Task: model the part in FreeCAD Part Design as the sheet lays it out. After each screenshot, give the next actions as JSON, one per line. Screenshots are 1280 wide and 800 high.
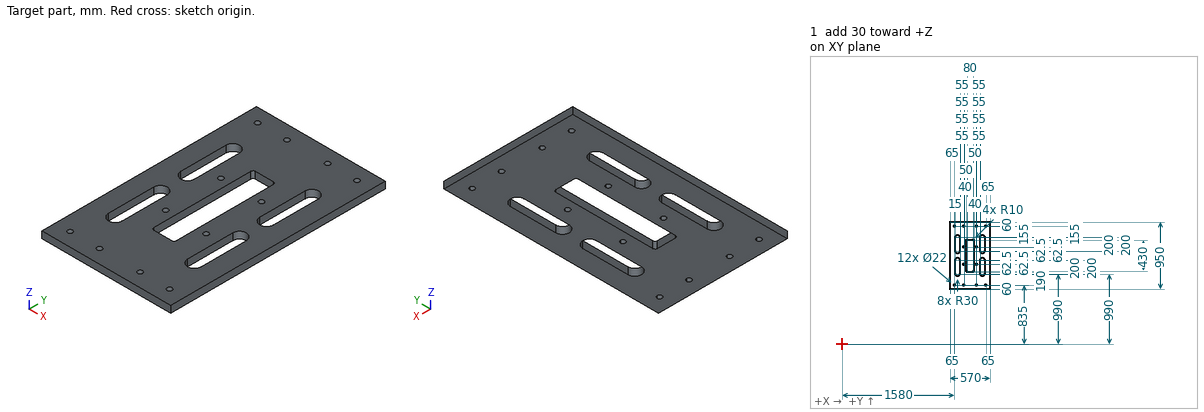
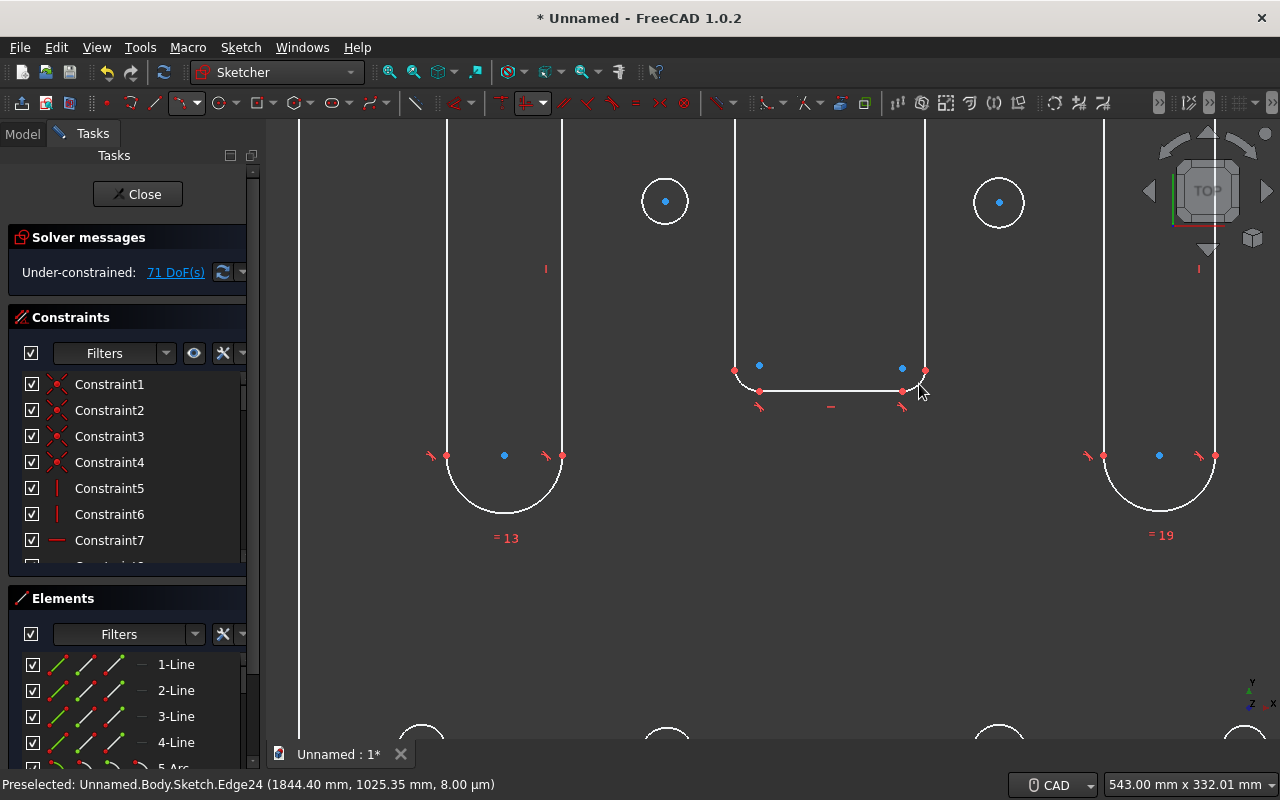
{"action": "scroll", "coordinate": [906, 388], "scroll_direction": "down", "scroll_amount": 10}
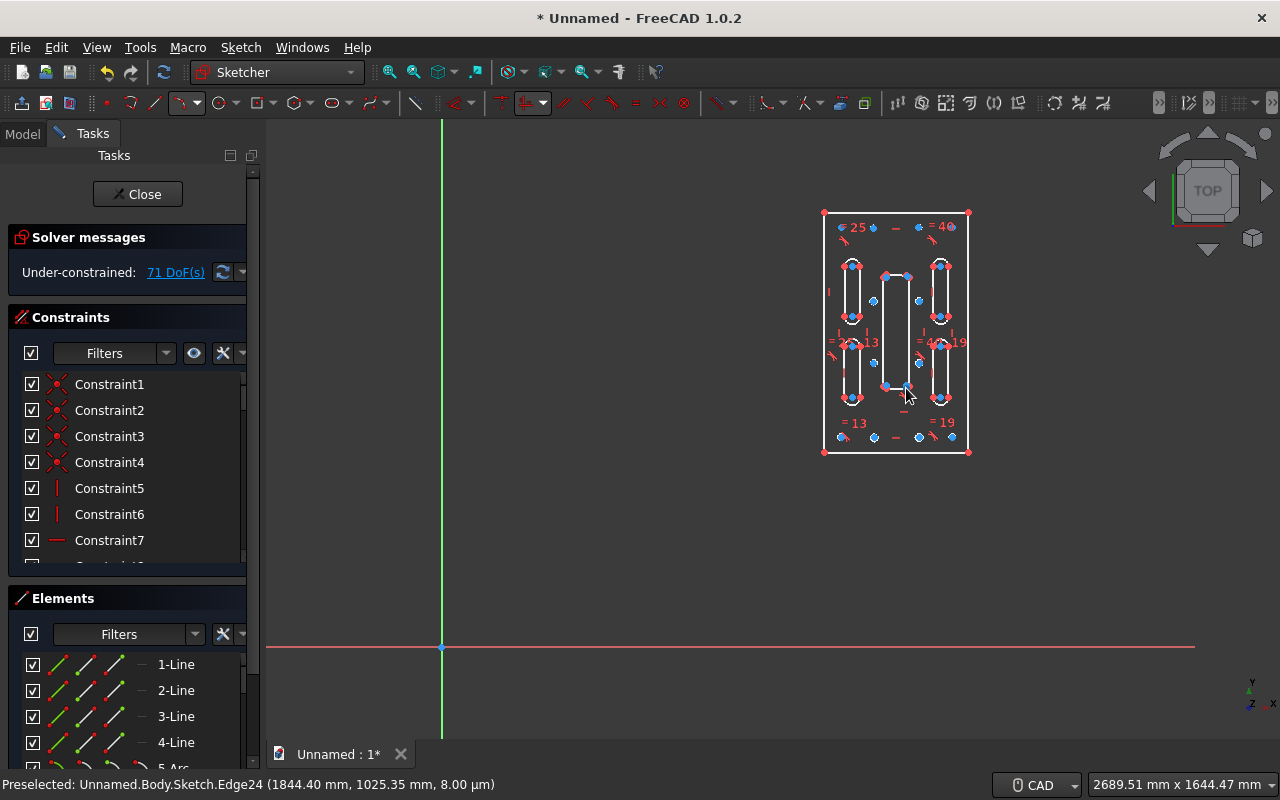
{"action": "scroll", "coordinate": [883, 364], "scroll_direction": "up", "scroll_amount": 4}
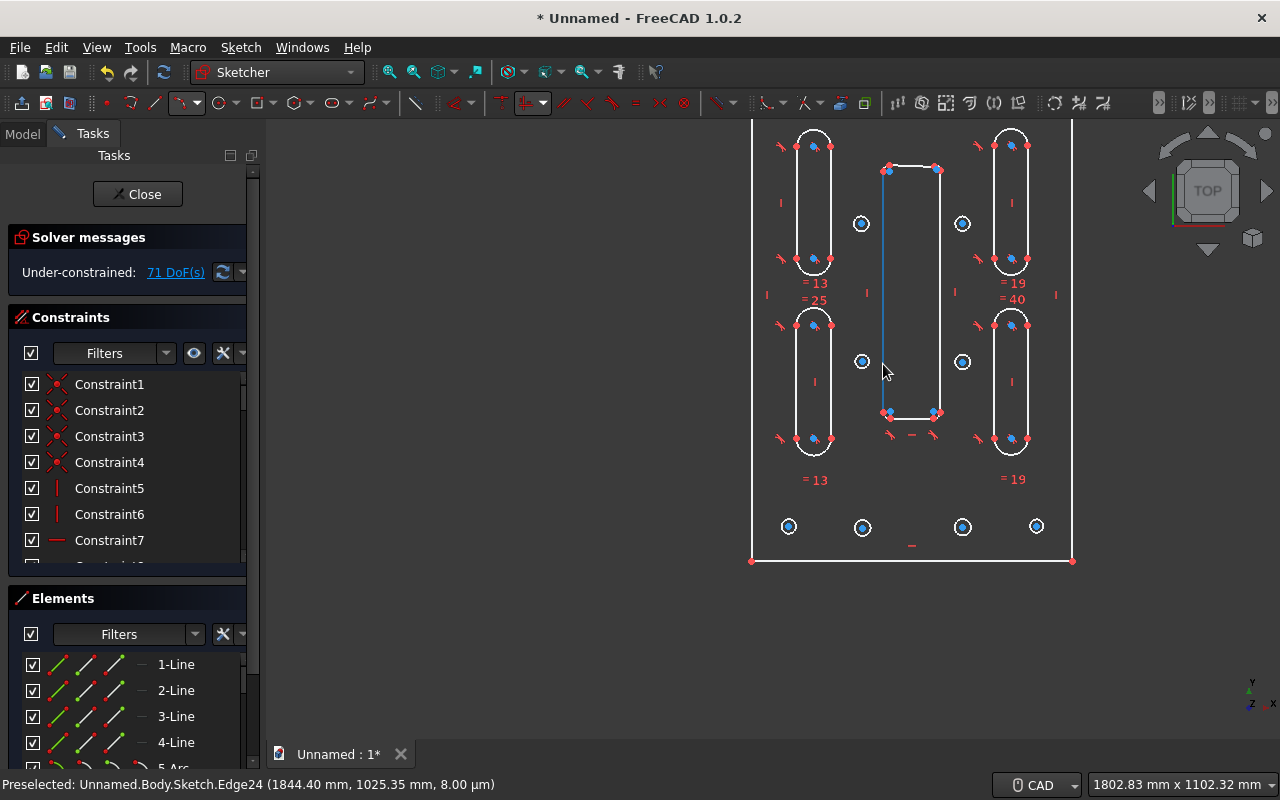
{"action": "left_click", "coordinate": [883, 364]}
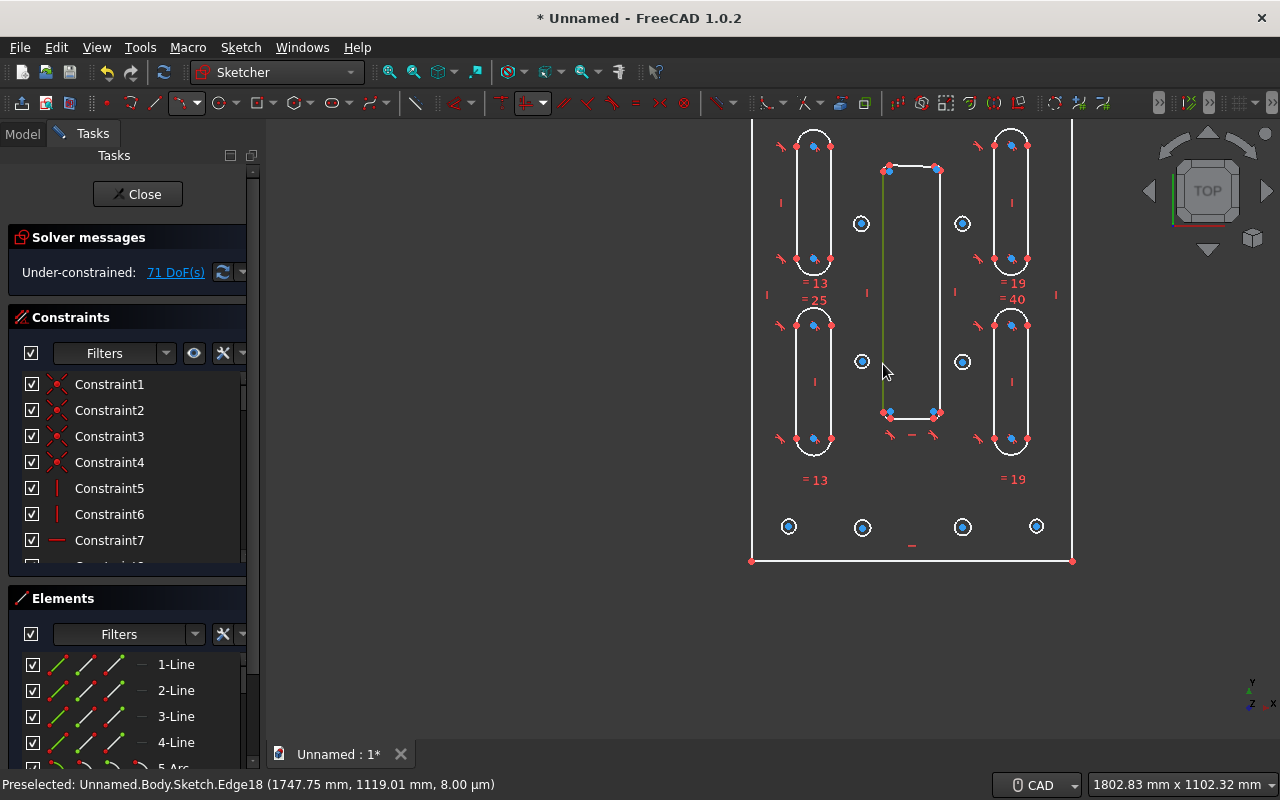
{"action": "scroll", "coordinate": [886, 417], "scroll_direction": "up", "scroll_amount": 5}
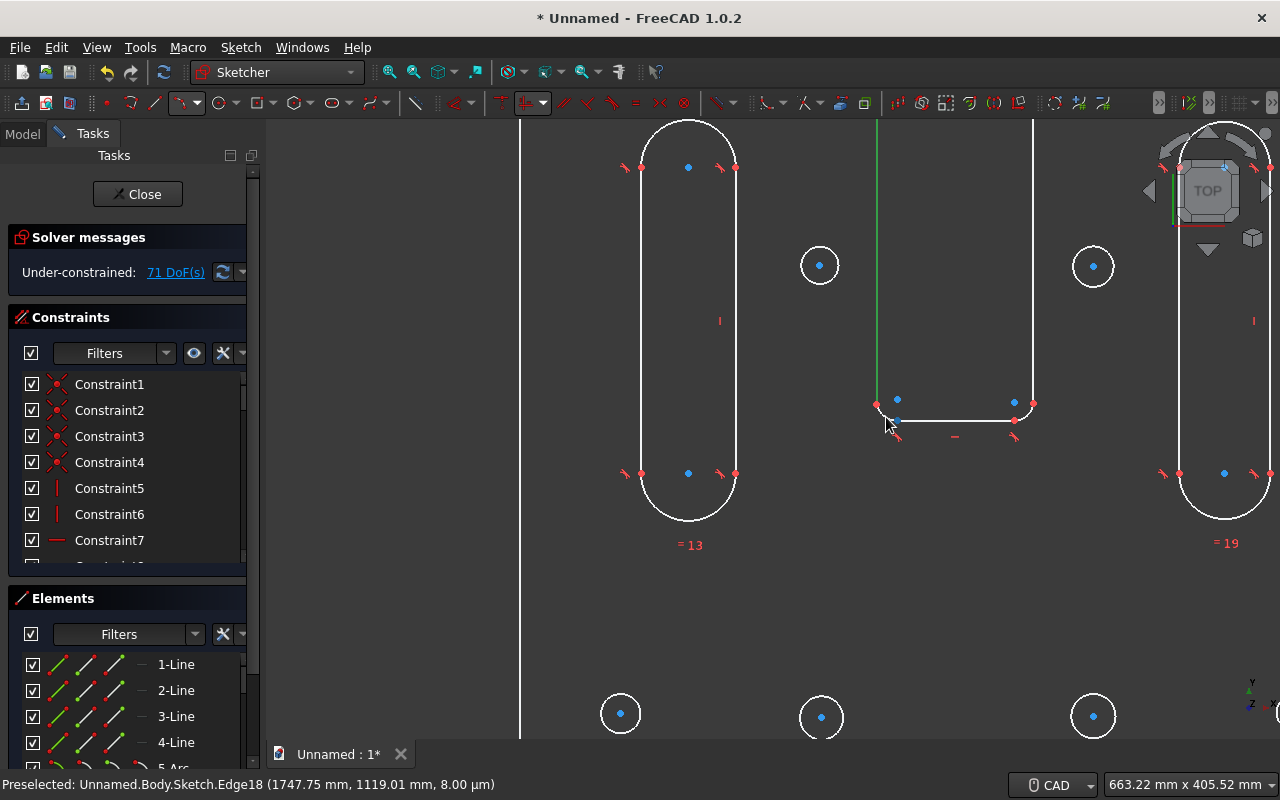
{"action": "left_click", "coordinate": [884, 416]}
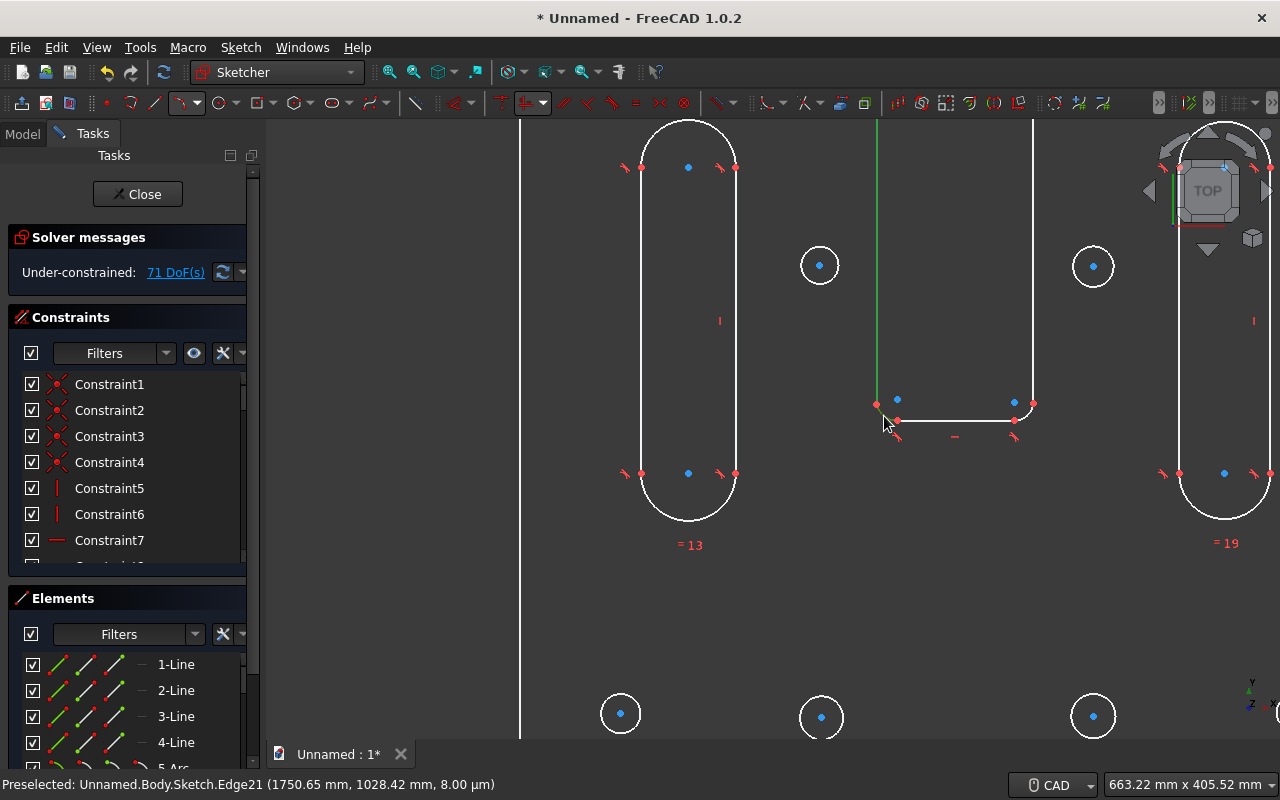
{"action": "left_click", "coordinate": [612, 104]}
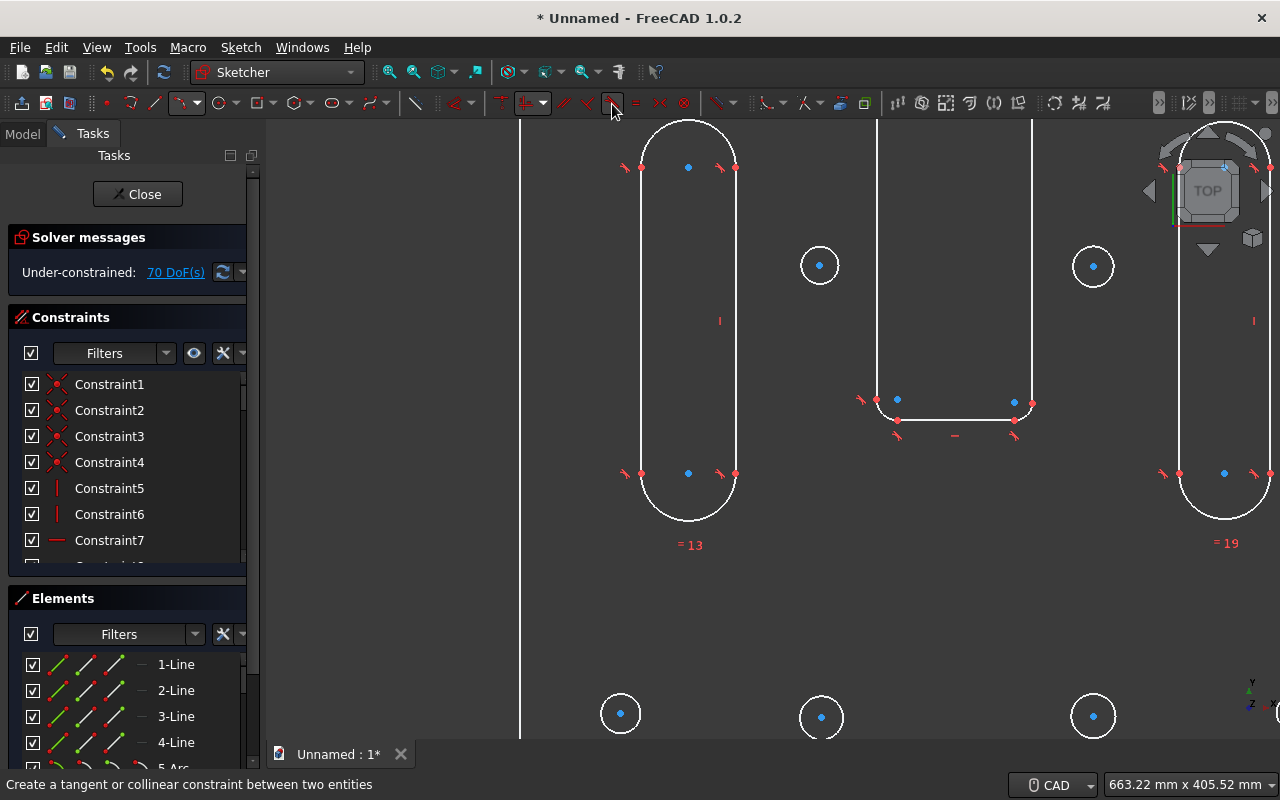
{"action": "scroll", "coordinate": [884, 382], "scroll_direction": "down", "scroll_amount": 9}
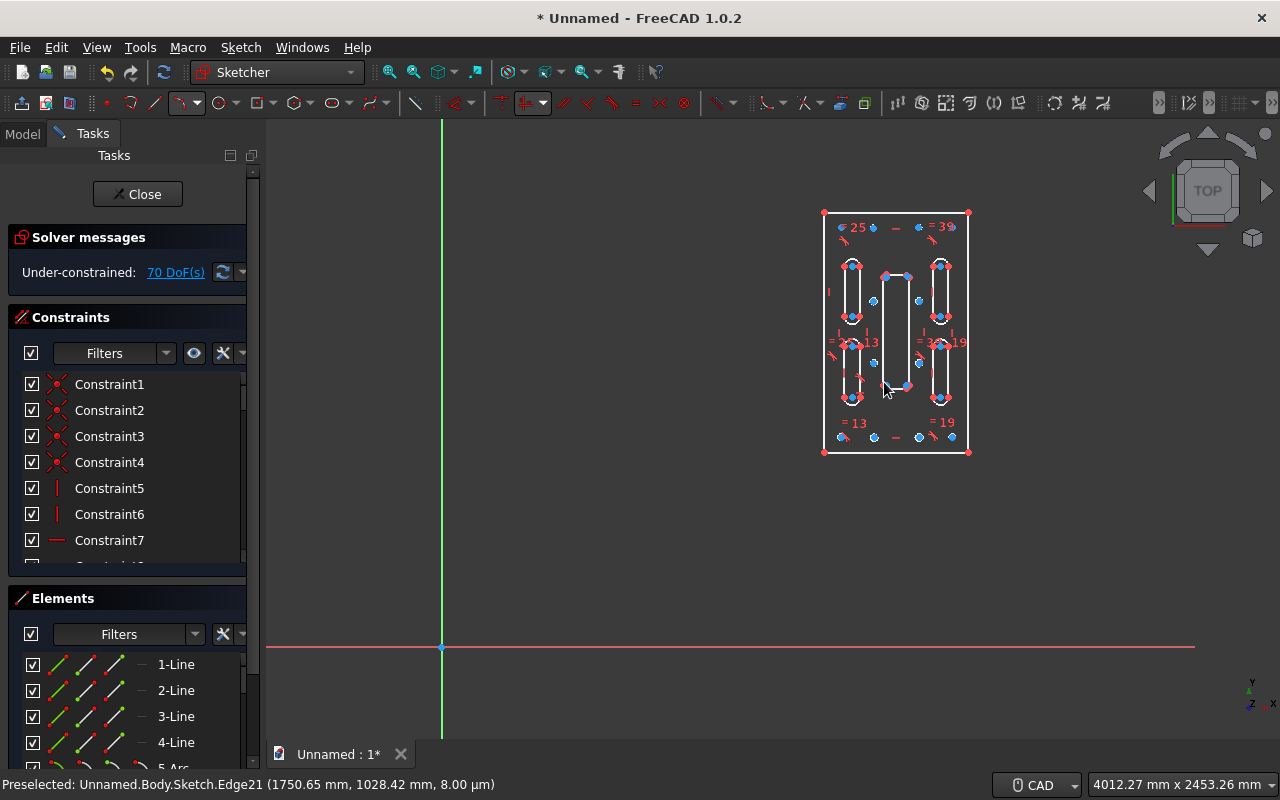
{"action": "scroll", "coordinate": [883, 353], "scroll_direction": "up", "scroll_amount": 2}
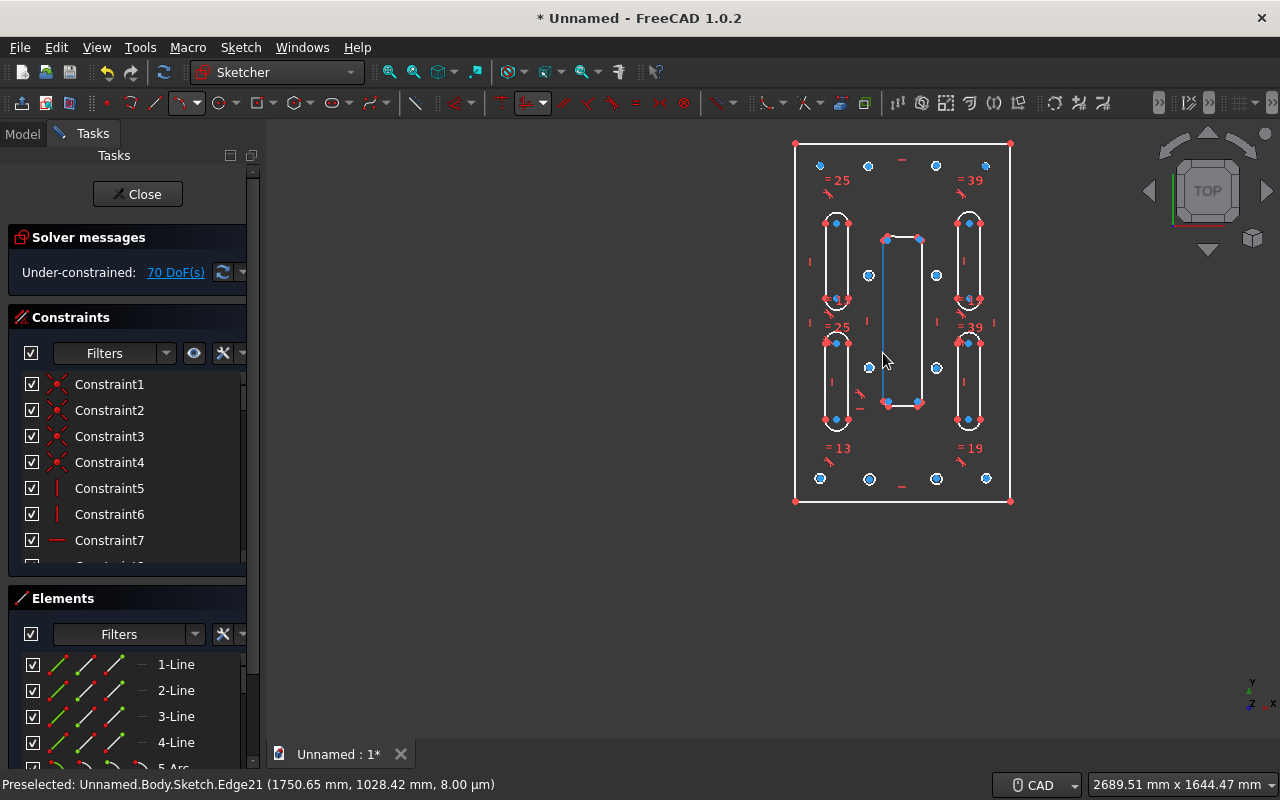
{"action": "left_click", "coordinate": [883, 353]}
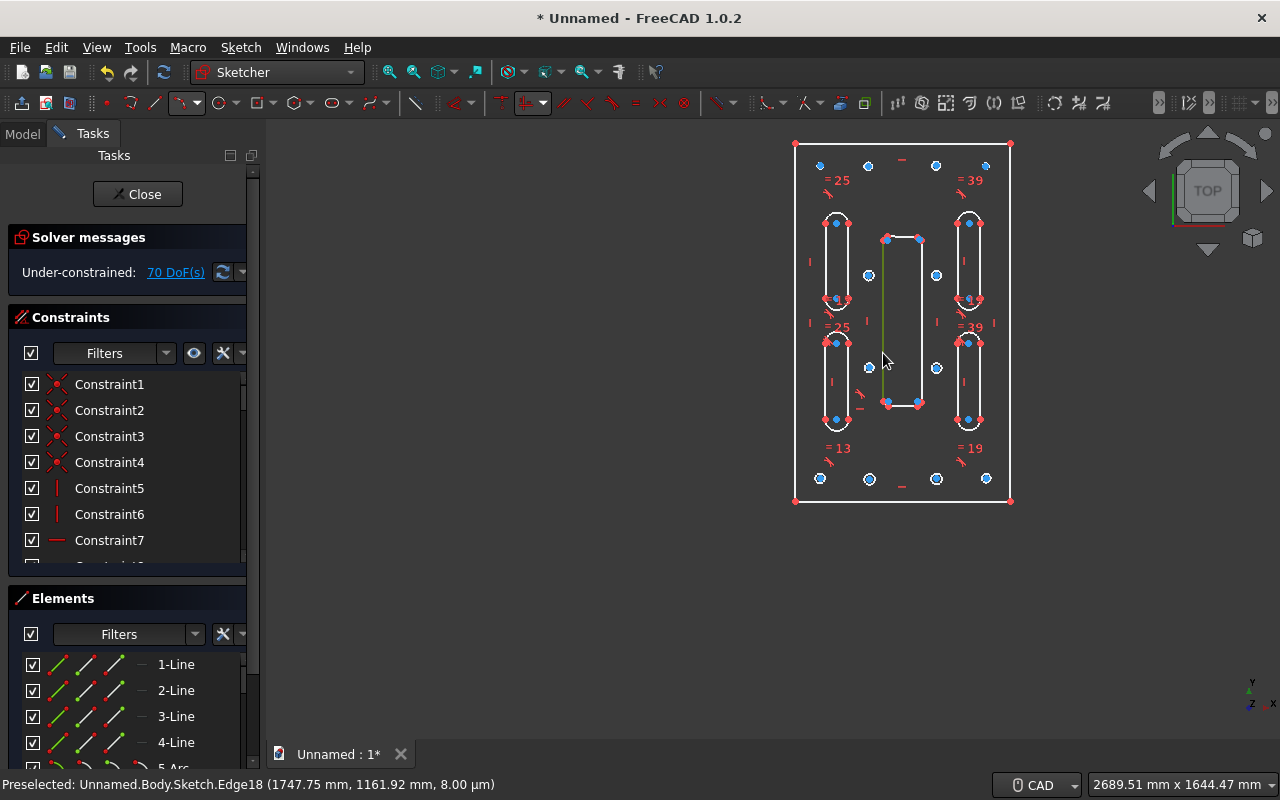
{"action": "scroll", "coordinate": [884, 237], "scroll_direction": "up", "scroll_amount": 7}